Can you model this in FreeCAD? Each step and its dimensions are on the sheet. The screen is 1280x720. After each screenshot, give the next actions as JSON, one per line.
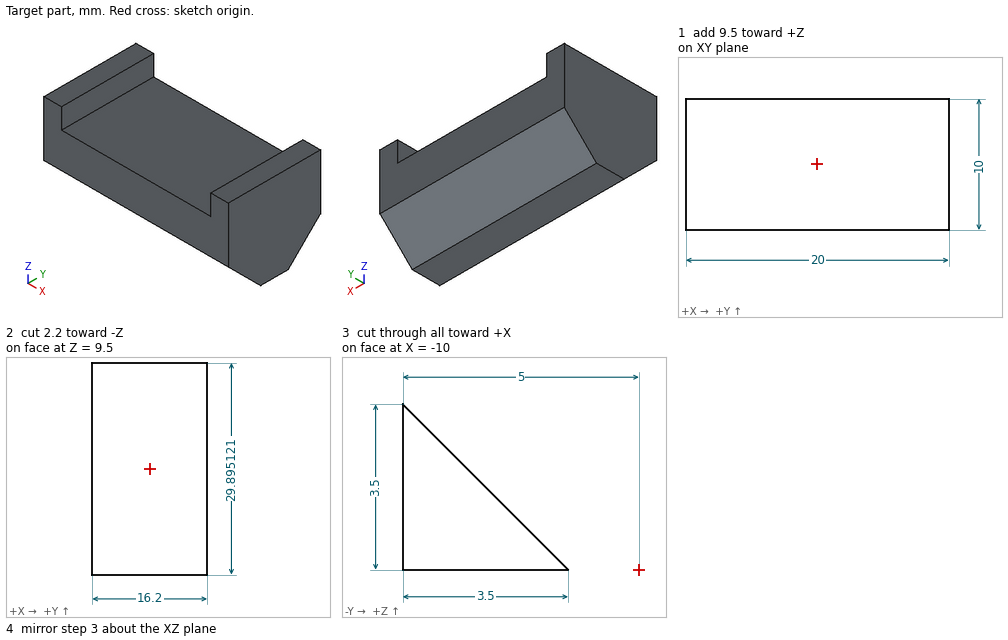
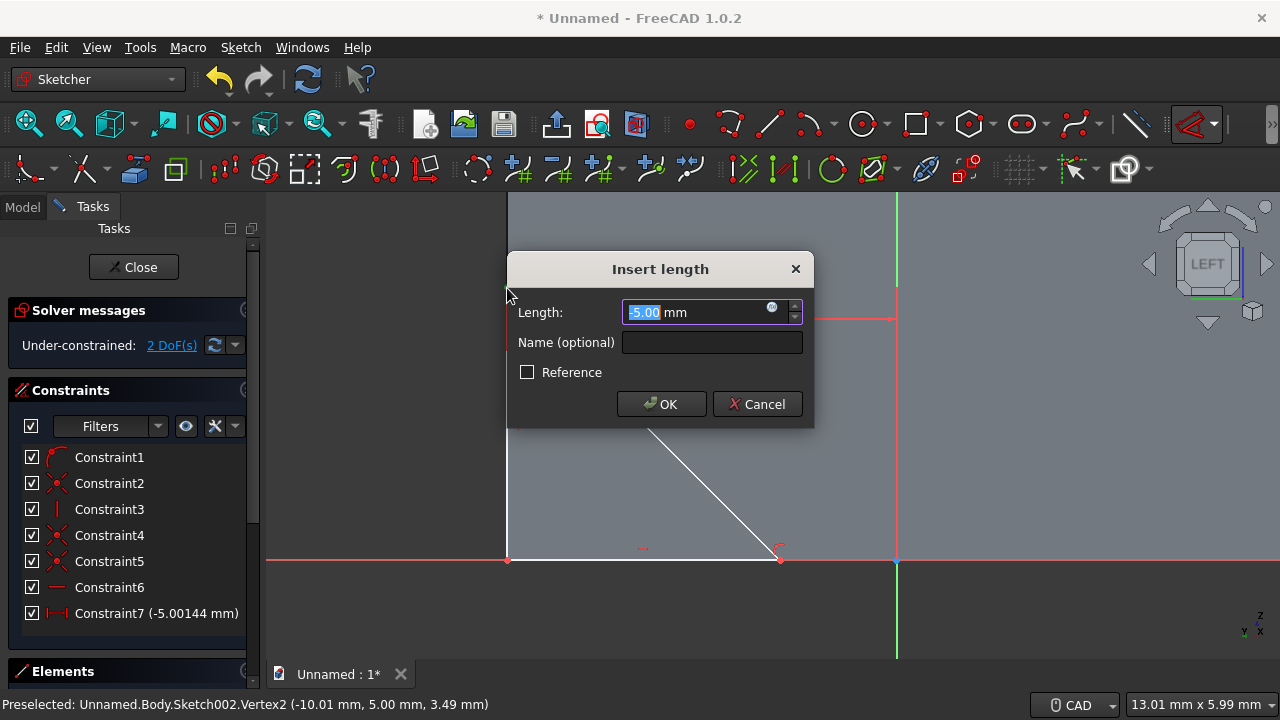
{"action": "type", "text": "-5"}
{"action": "key", "text": "Return"}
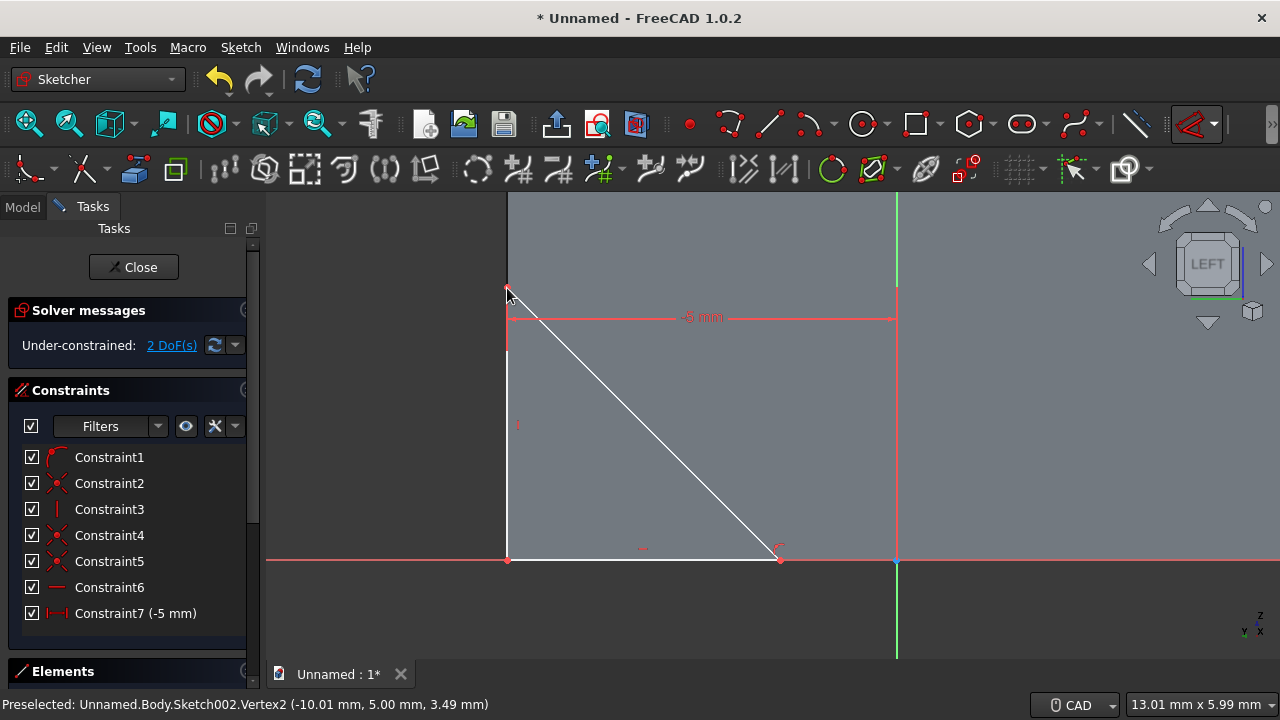
{"action": "left_click", "coordinate": [507, 370]}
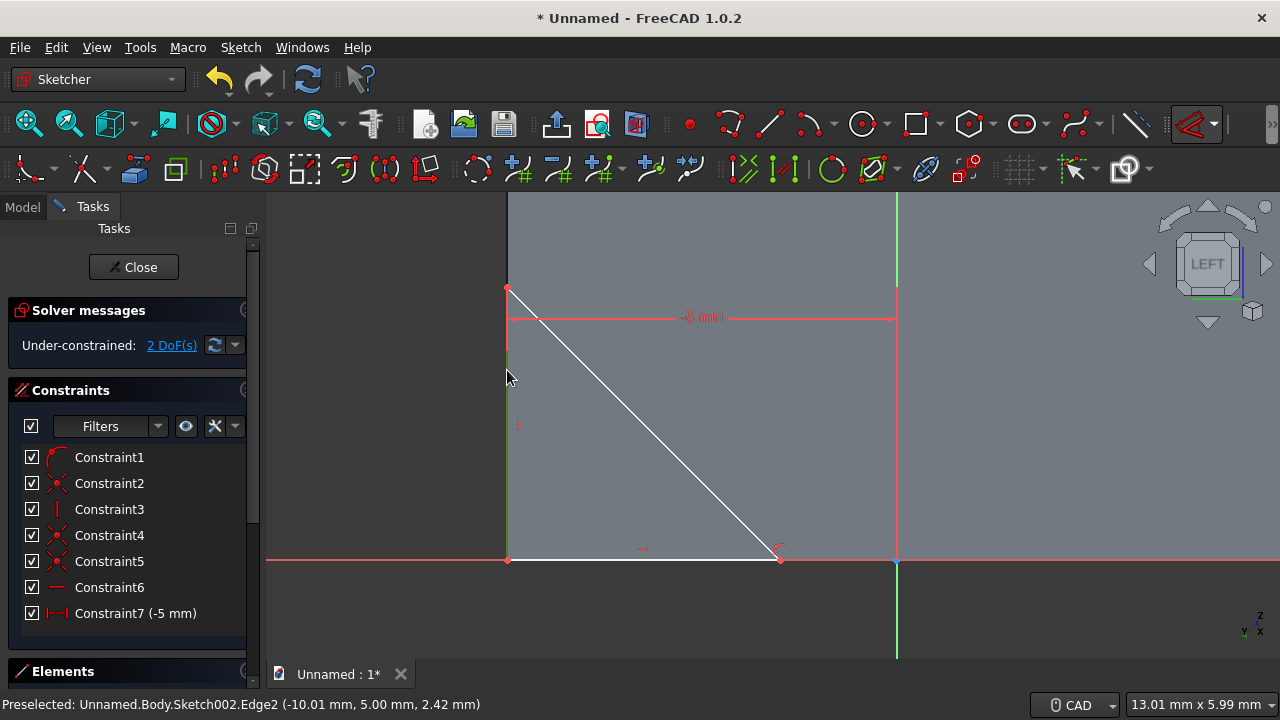
{"action": "key", "text": "i"}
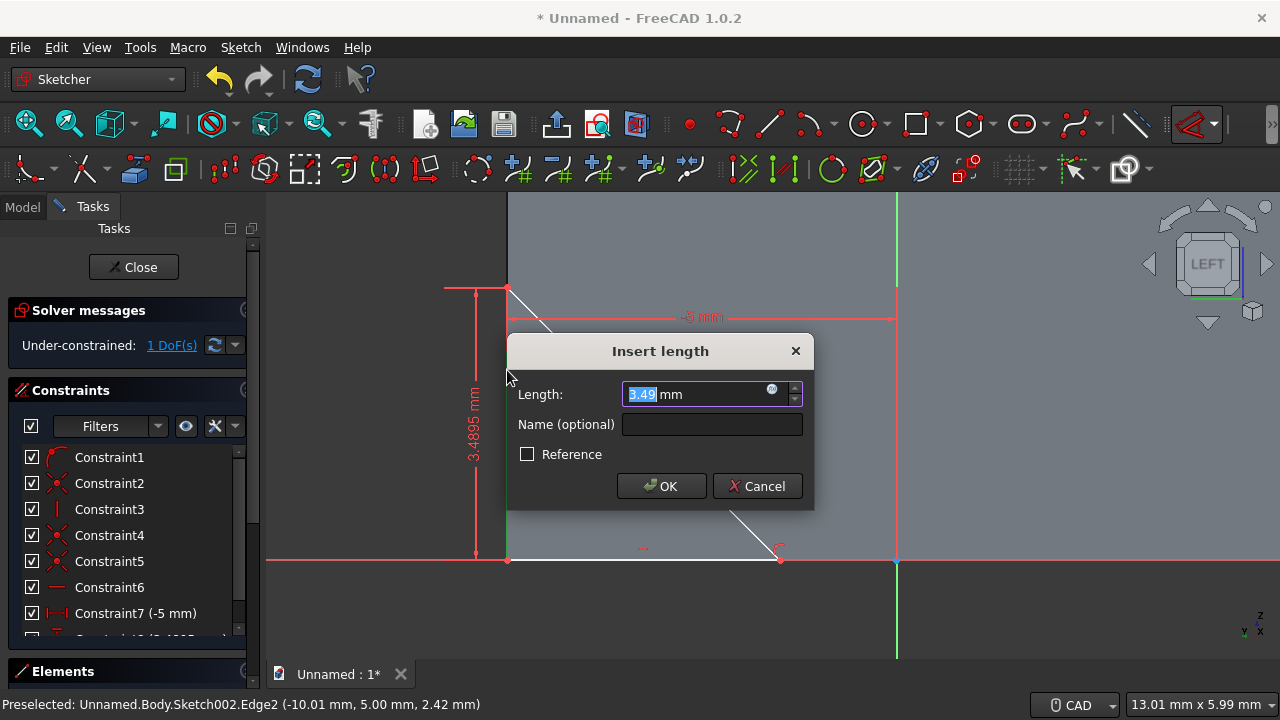
{"action": "type", "text": "3.5"}
{"action": "key", "text": "Return"}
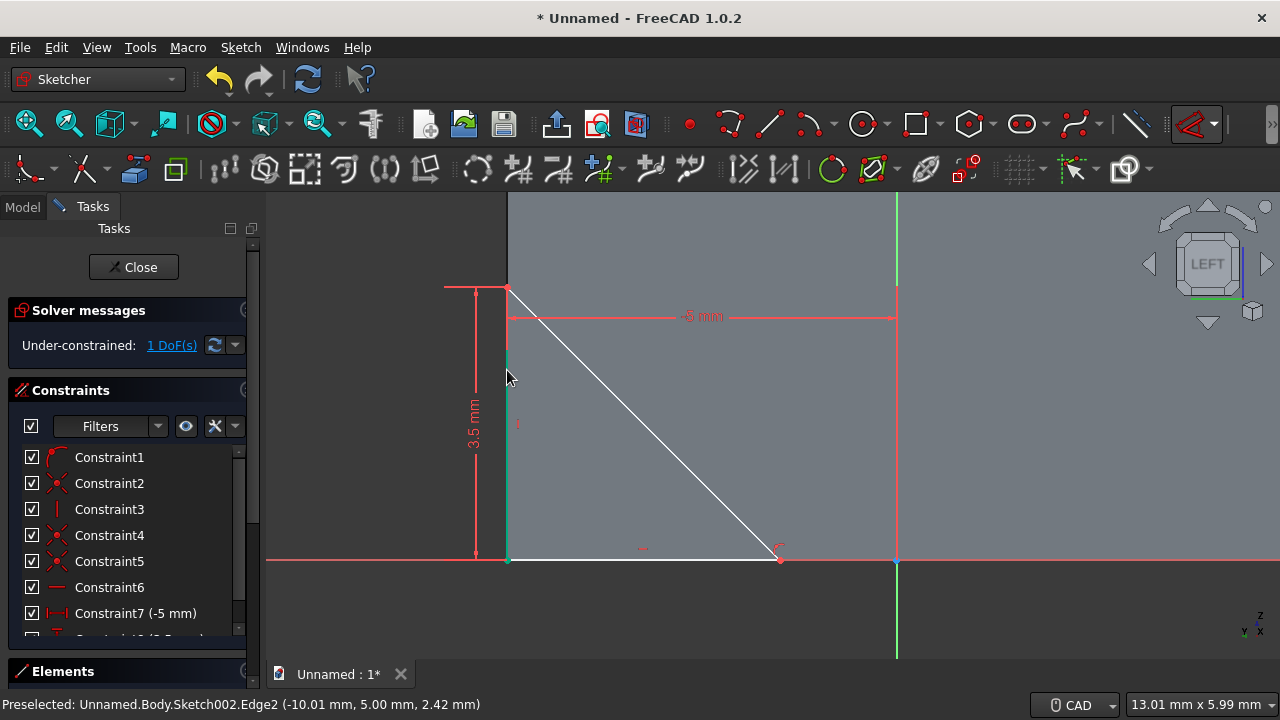
{"action": "left_click", "coordinate": [589, 560]}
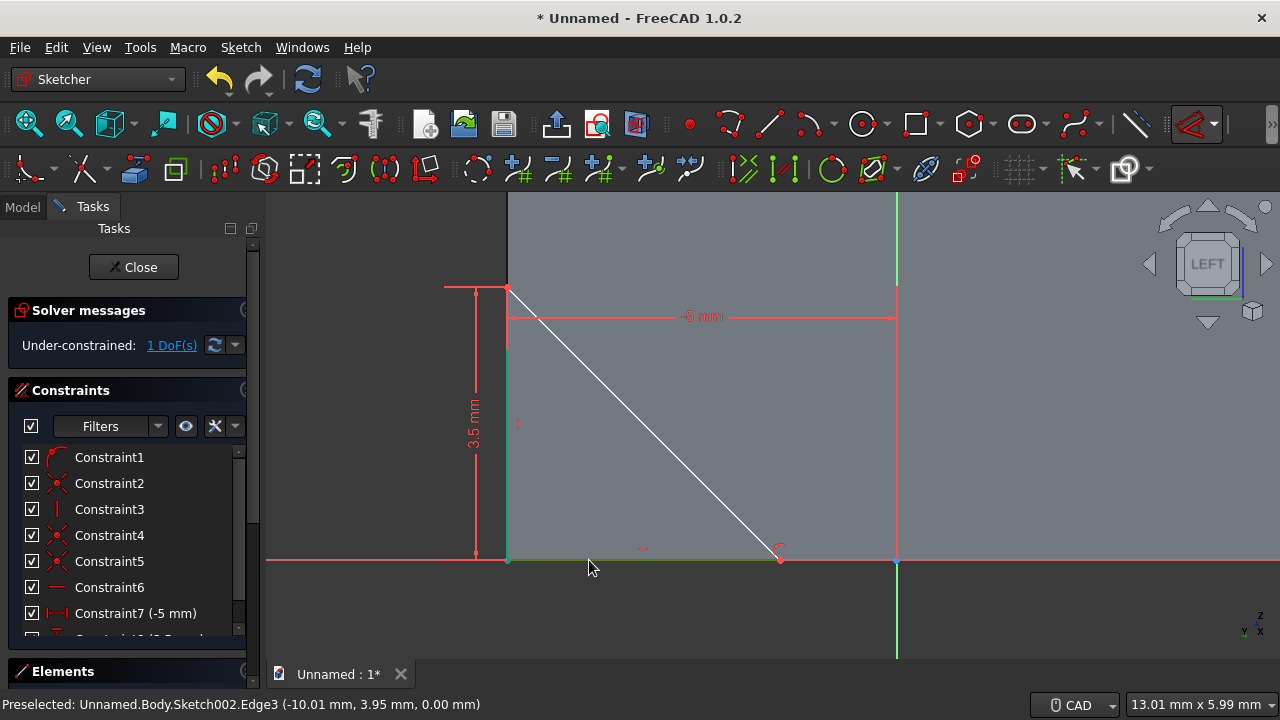
{"action": "left_click", "coordinate": [1216, 124]}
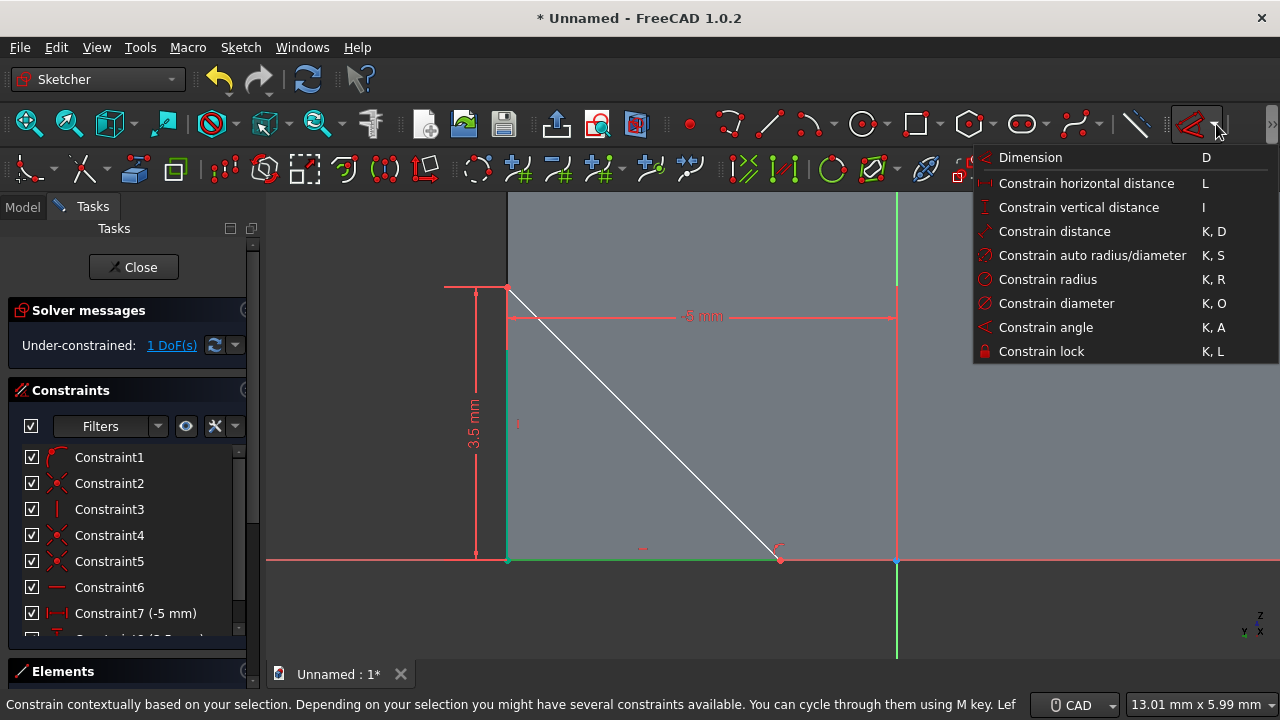
{"action": "left_click", "coordinate": [1126, 183]}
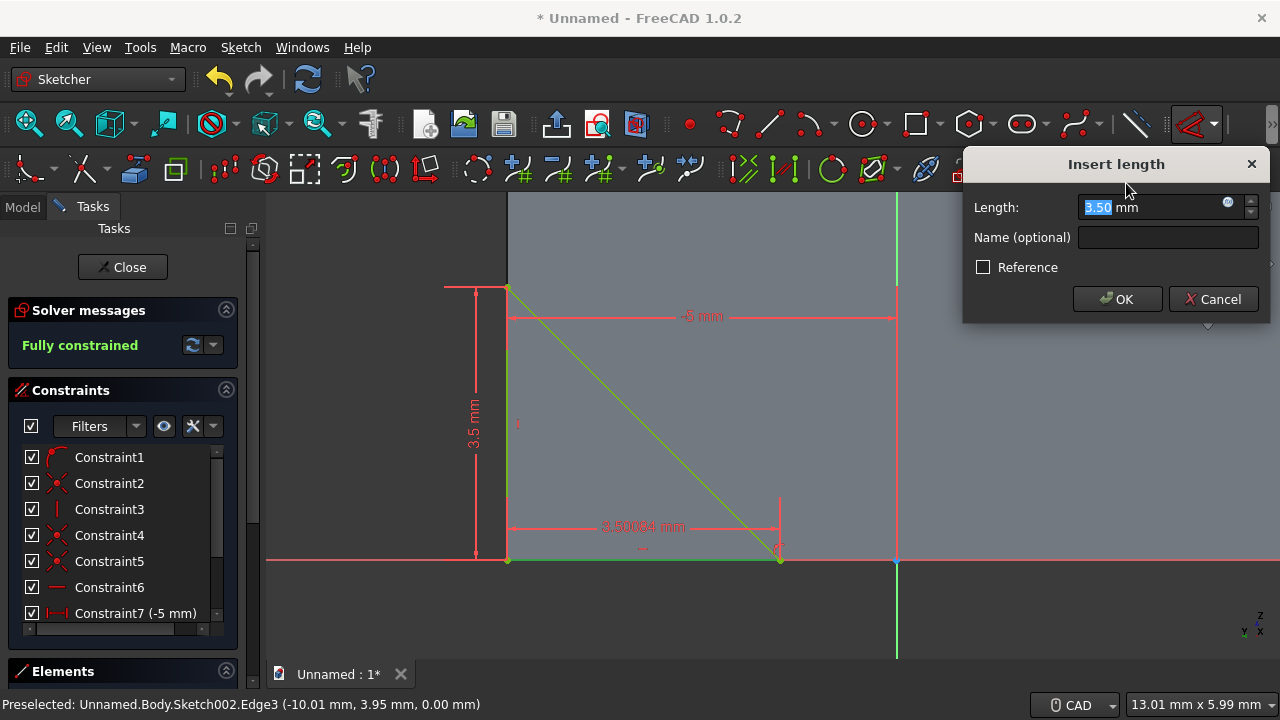
{"action": "type", "text": "3.5"}
{"action": "key", "text": "Return"}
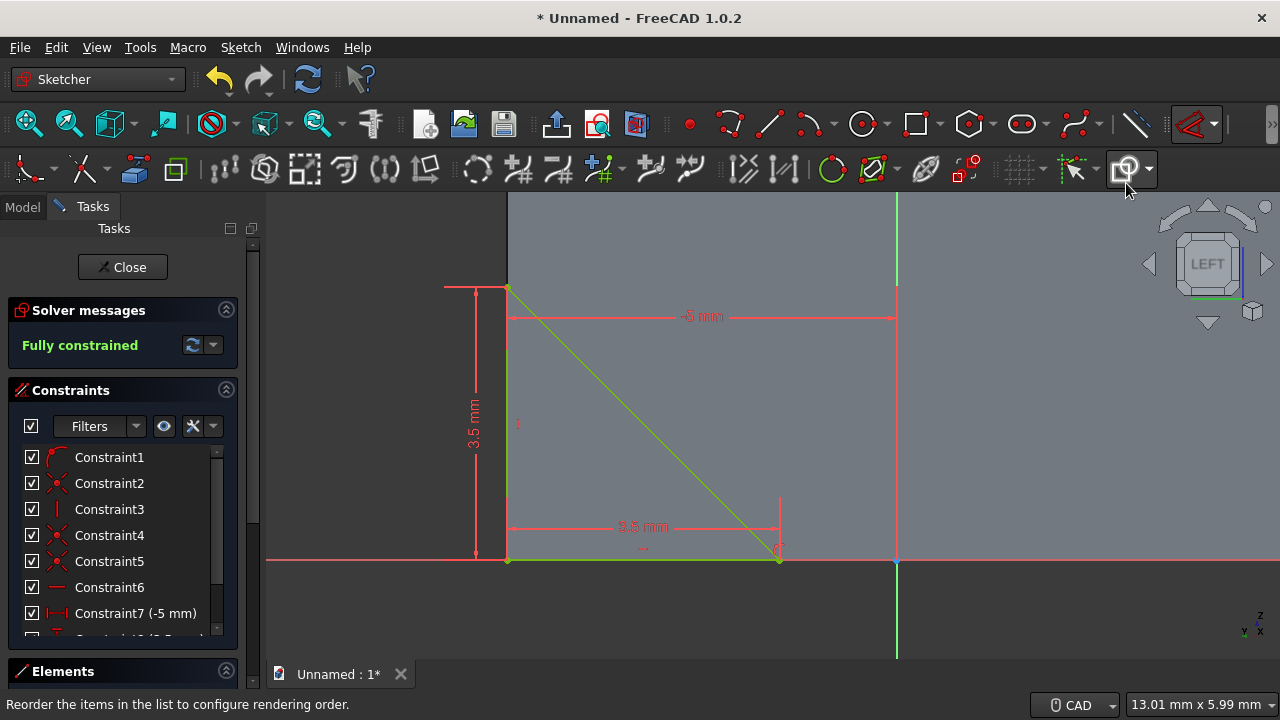
{"action": "left_click", "coordinate": [123, 267]}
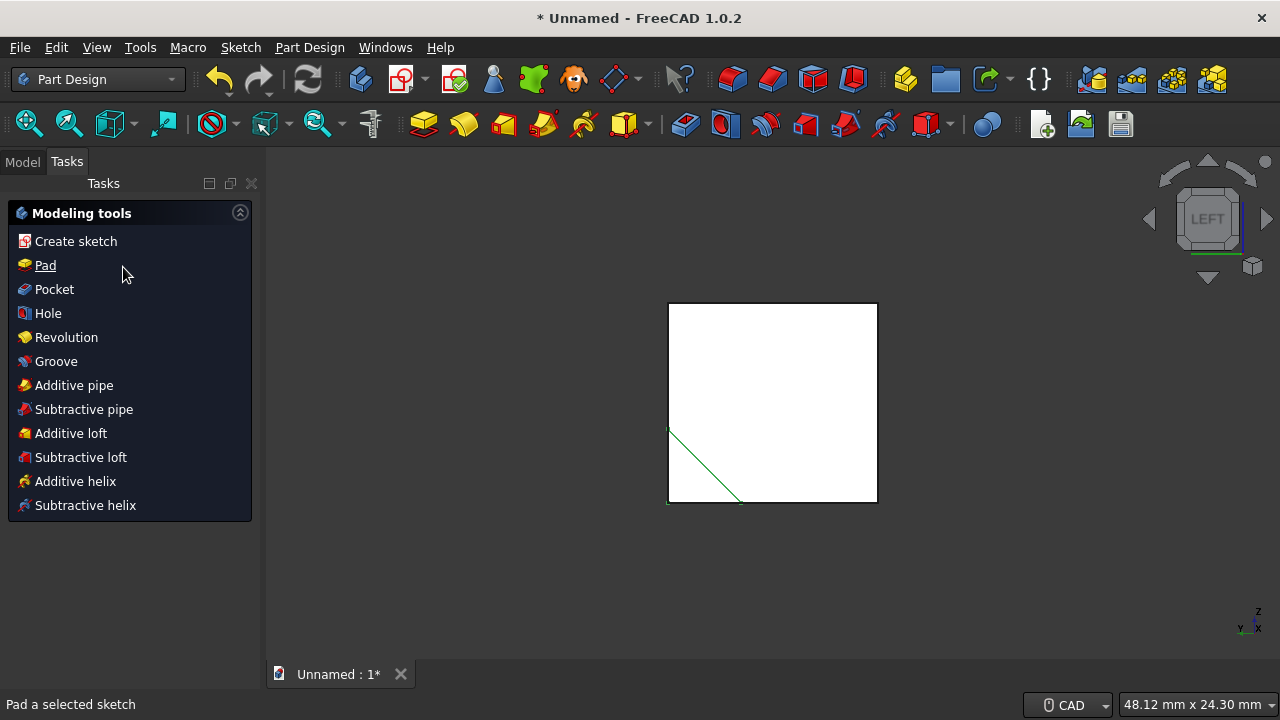
{"action": "left_click", "coordinate": [686, 124]}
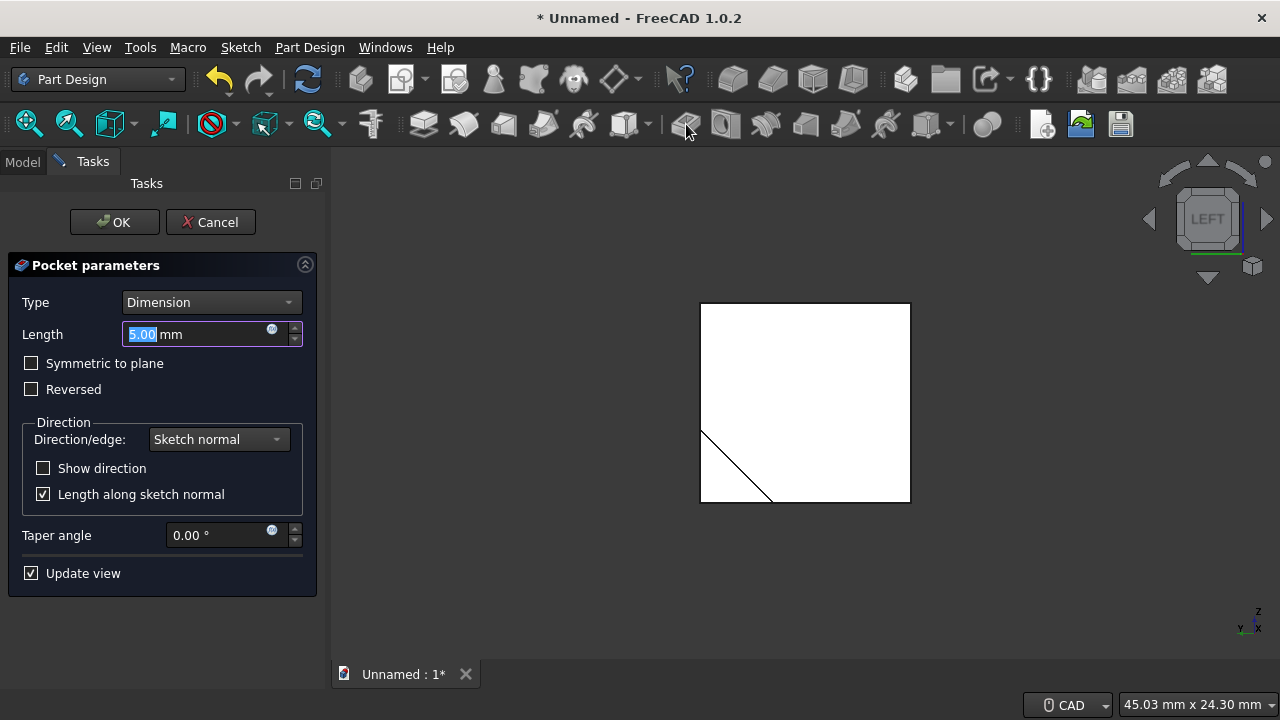
{"action": "left_click", "coordinate": [212, 302]}